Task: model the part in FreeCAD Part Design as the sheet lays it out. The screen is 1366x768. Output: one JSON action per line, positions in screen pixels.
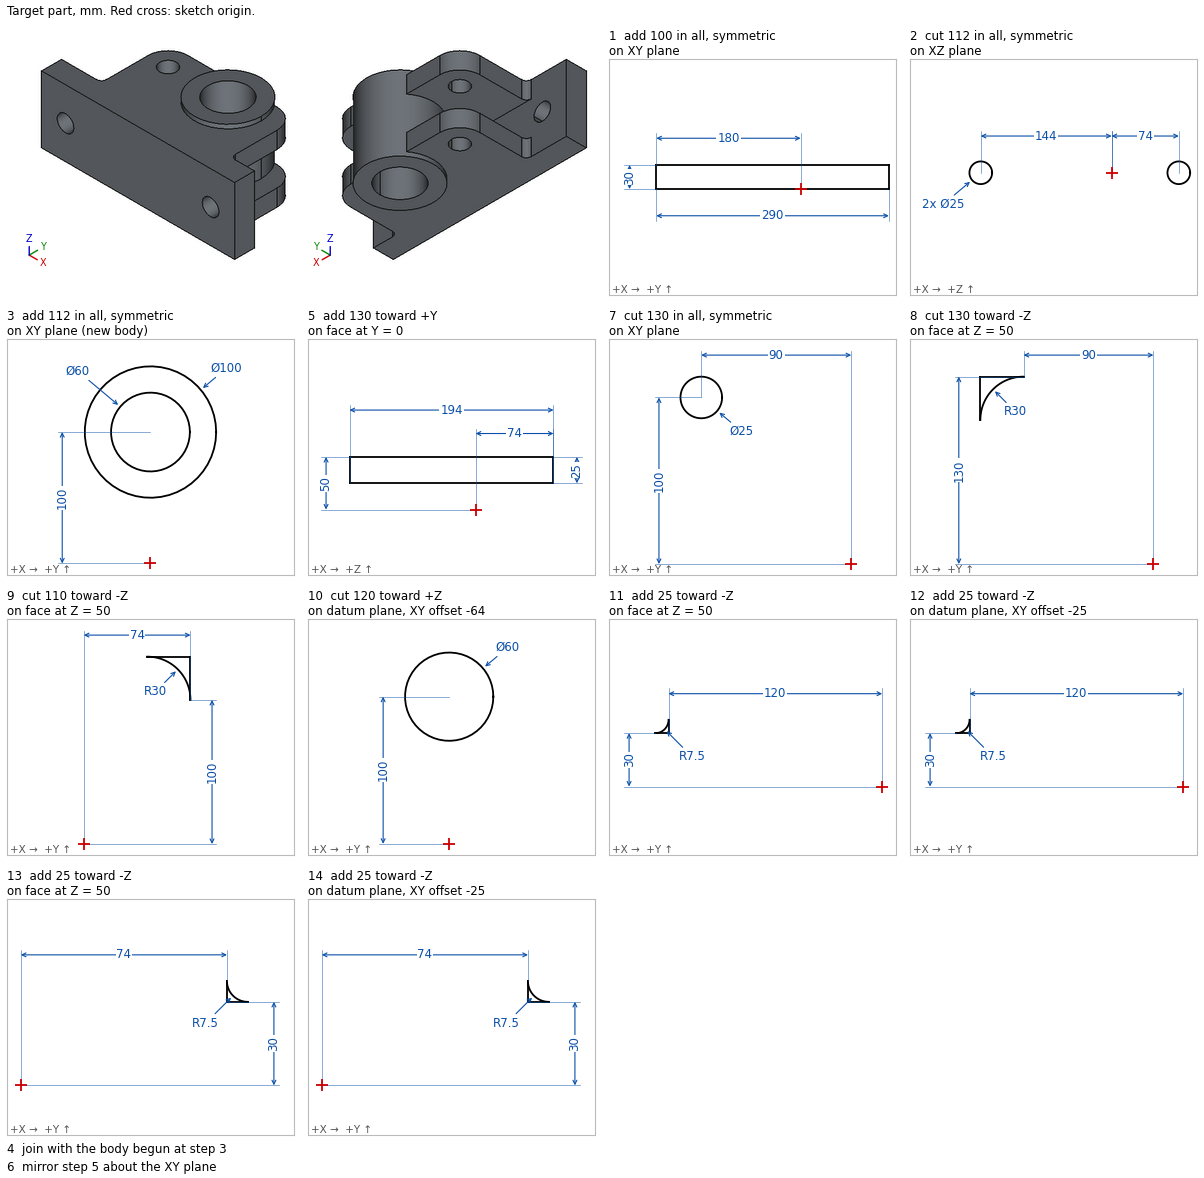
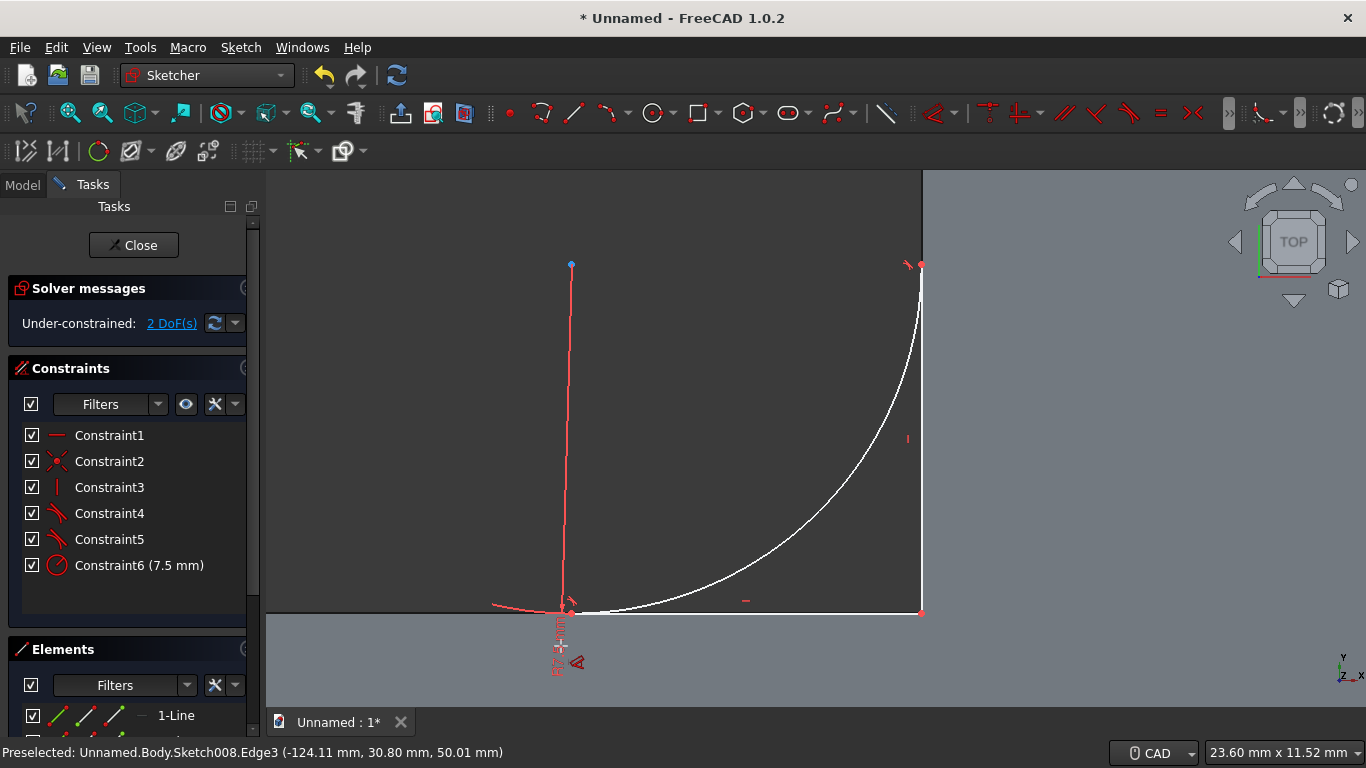
{"action": "left_click", "coordinate": [572, 614]}
{"action": "left_click", "coordinate": [538, 623]}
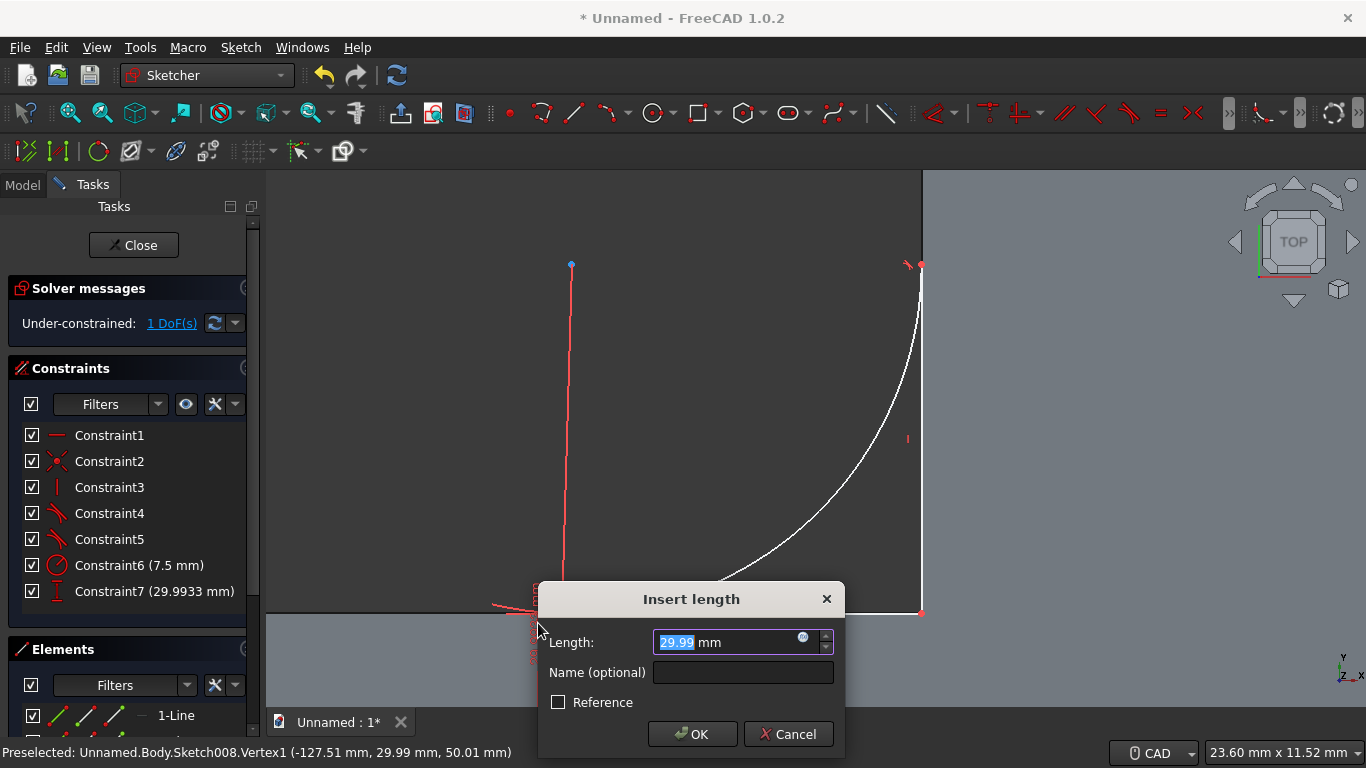
{"action": "type", "text": "30"}
{"action": "key", "text": "Return"}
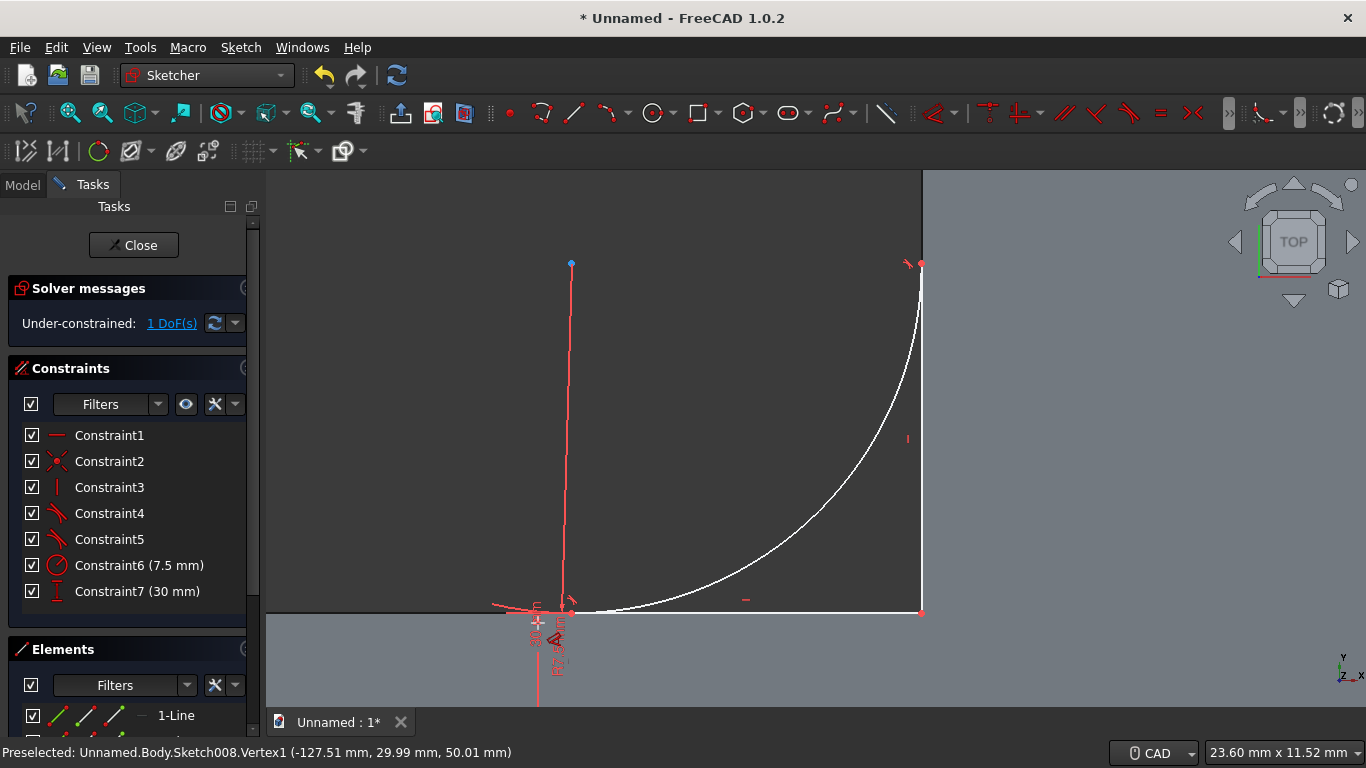
{"action": "left_click", "coordinate": [922, 613]}
{"action": "left_click", "coordinate": [1061, 579]}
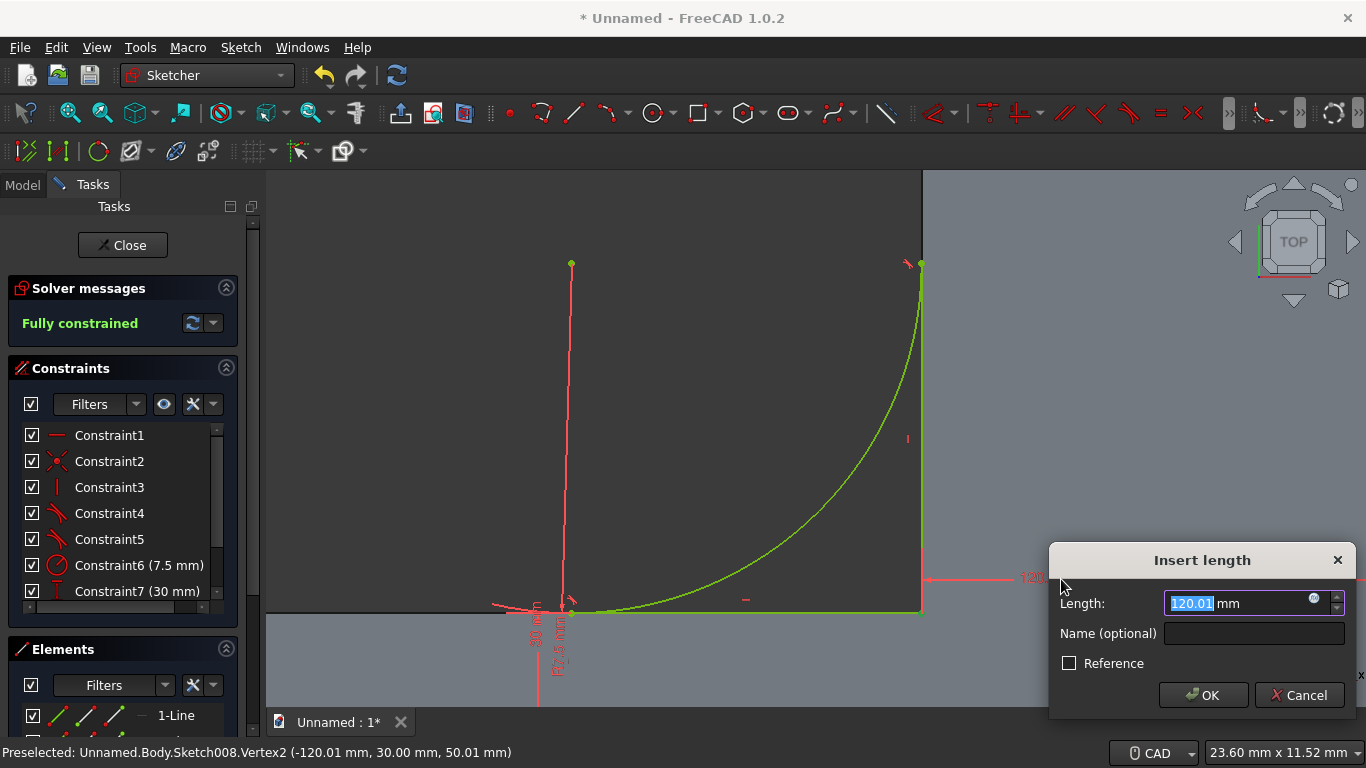
{"action": "type", "text": "120"}
{"action": "key", "text": "Return"}
{"action": "key", "text": "Escape"}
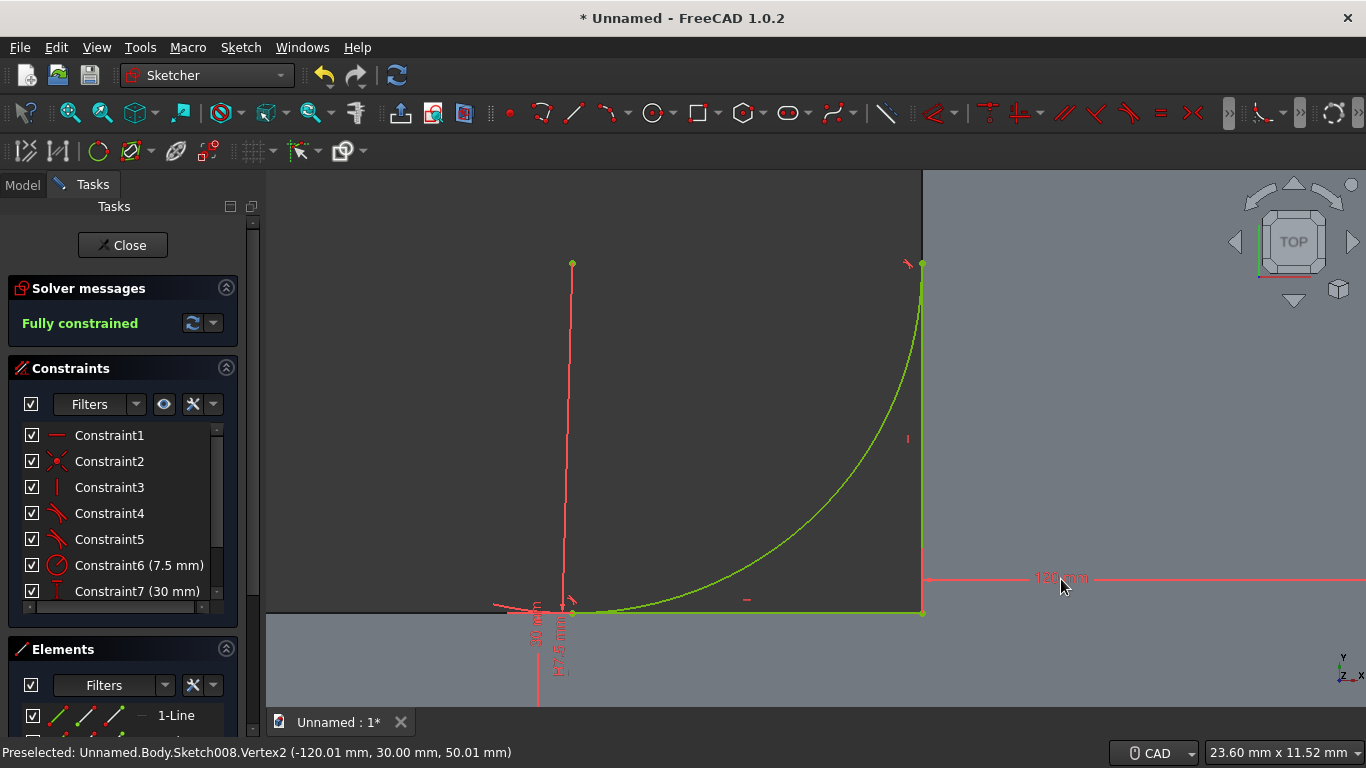
{"action": "left_click", "coordinate": [123, 245]}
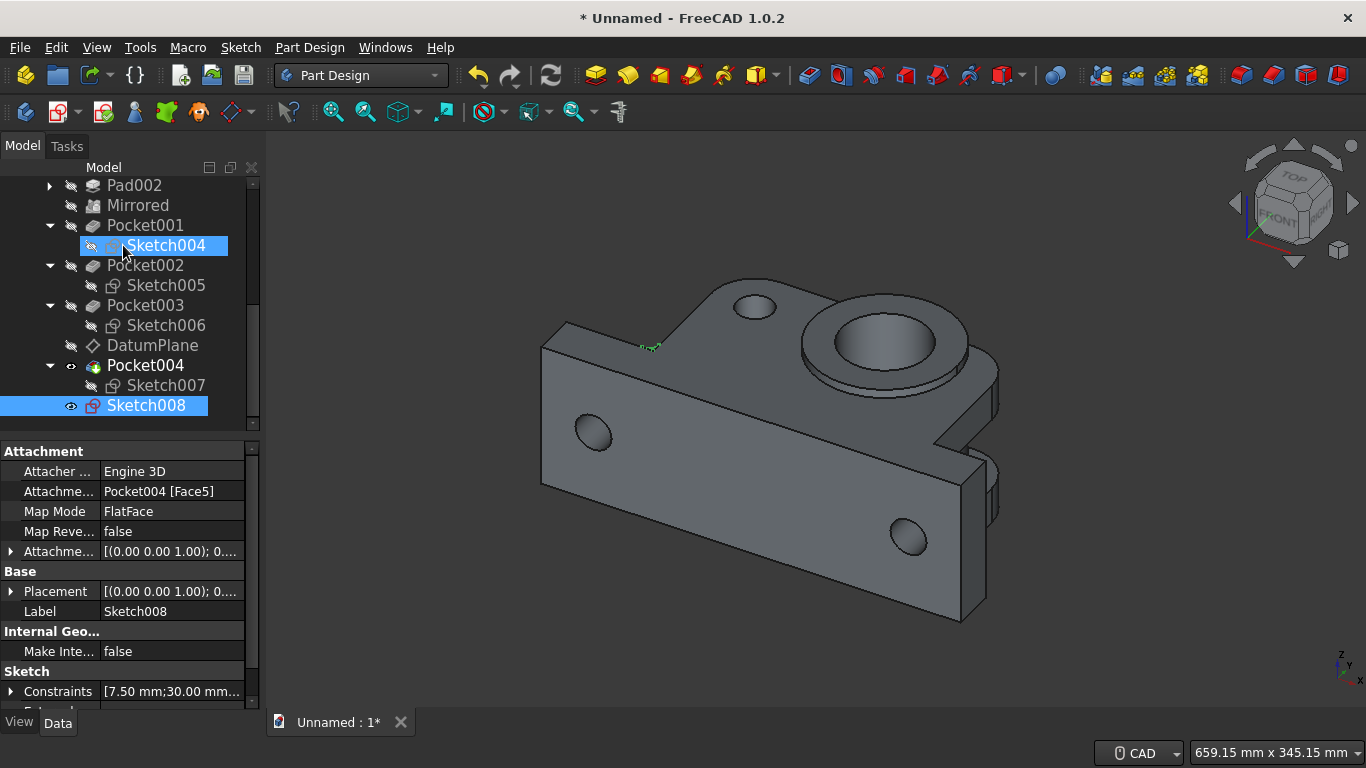
{"action": "left_click", "coordinate": [596, 76]}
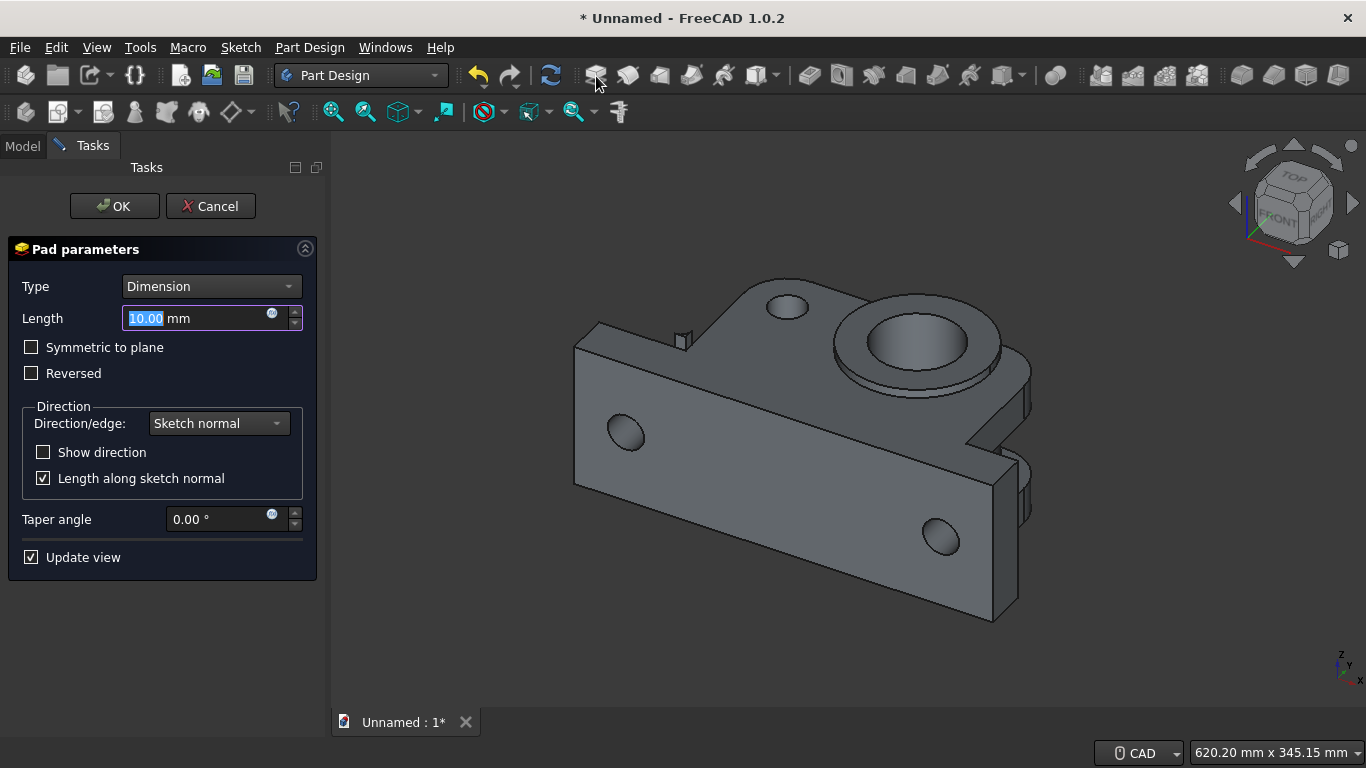
{"action": "type", "text": "25"}
{"action": "key", "text": "Tab"}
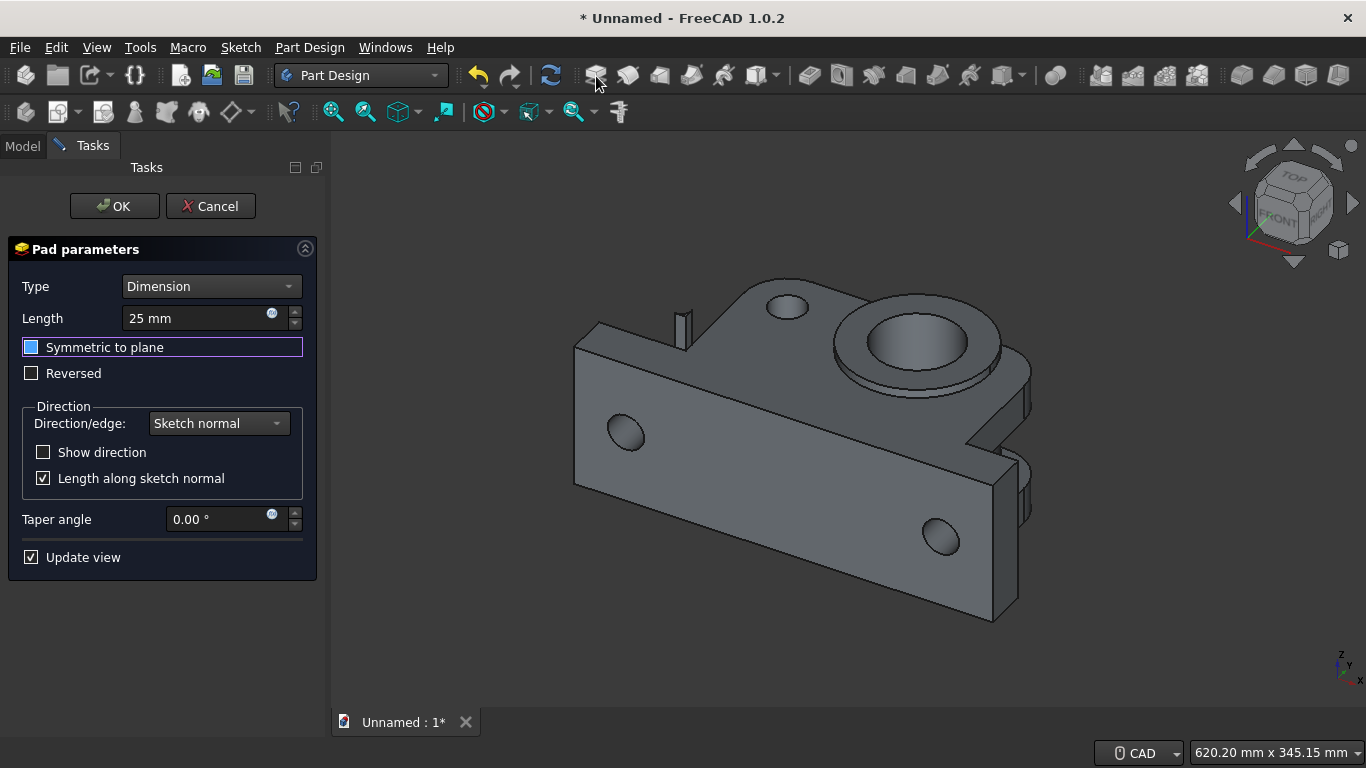
{"action": "left_click", "coordinate": [30, 373]}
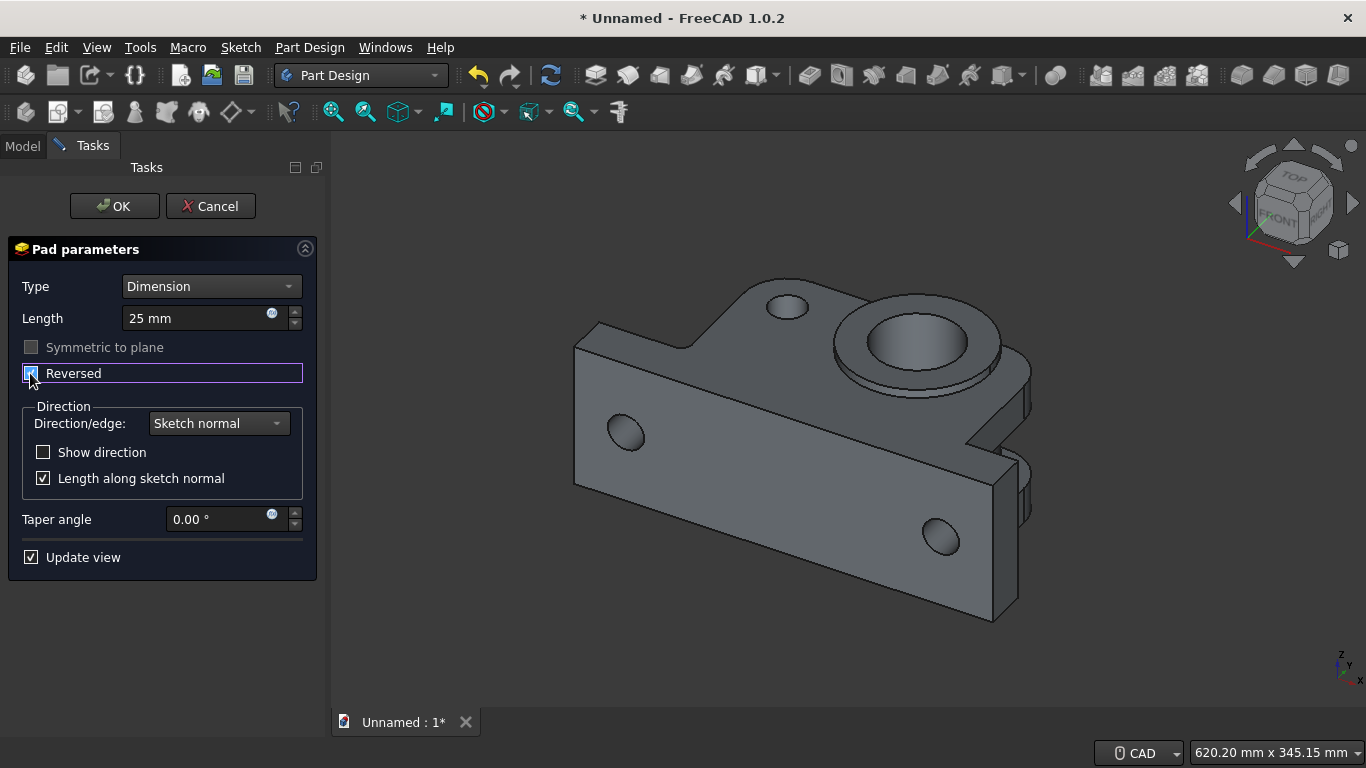
{"action": "left_click", "coordinate": [115, 206]}